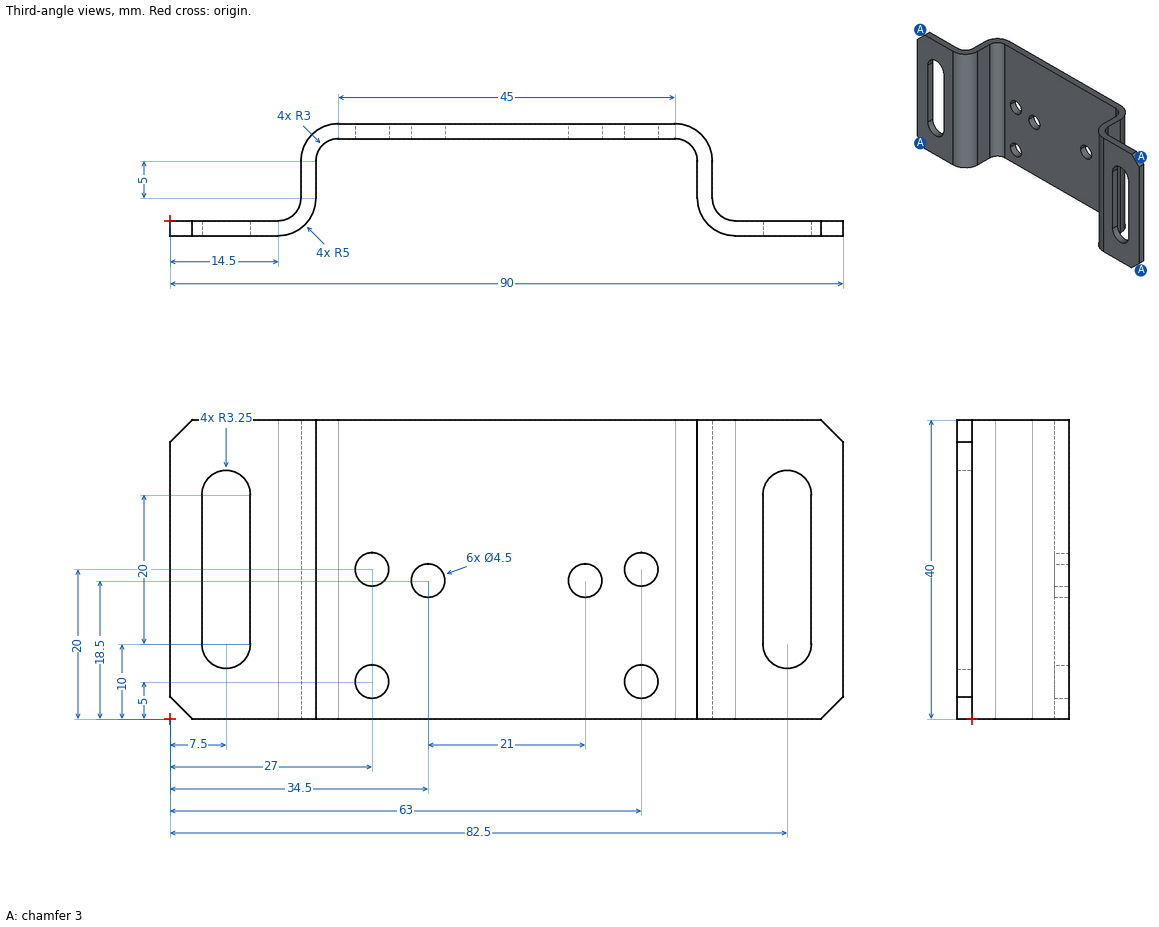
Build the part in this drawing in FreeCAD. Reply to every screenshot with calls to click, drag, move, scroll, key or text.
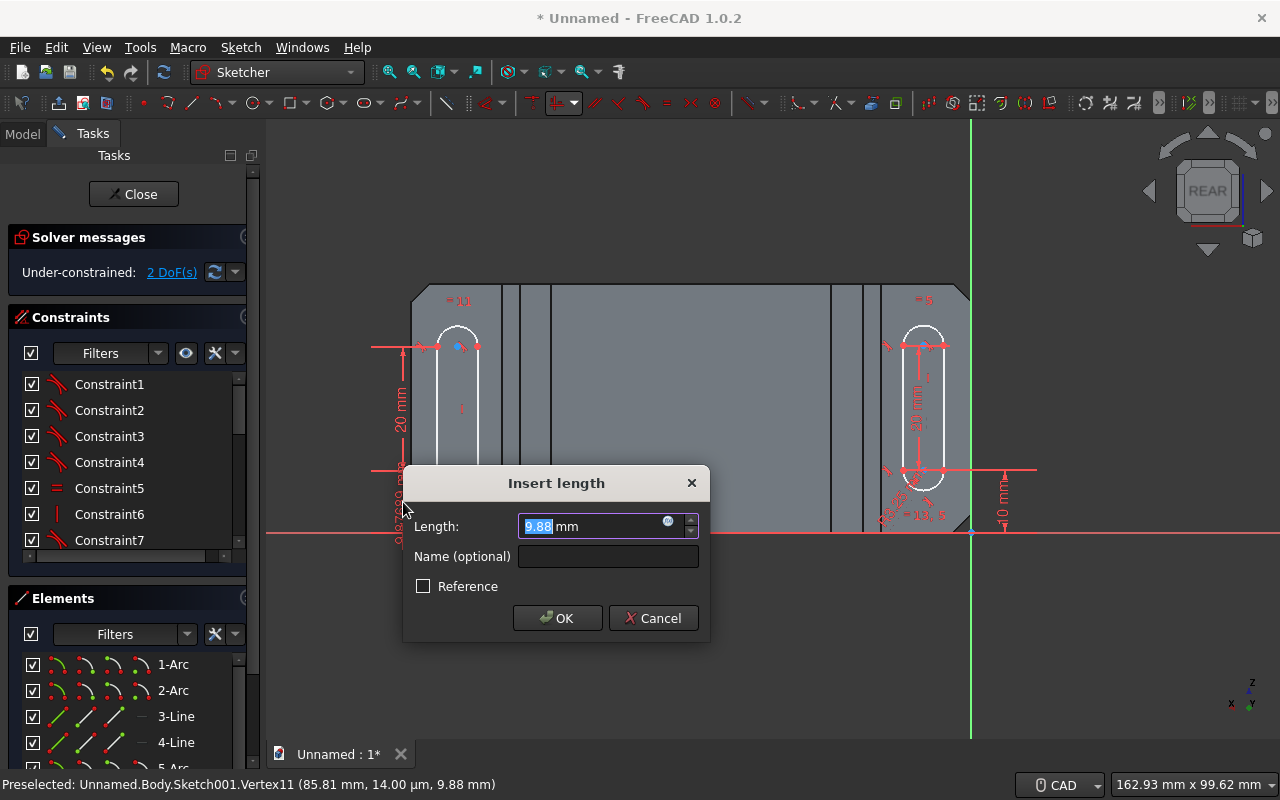
text(10)
key(Return)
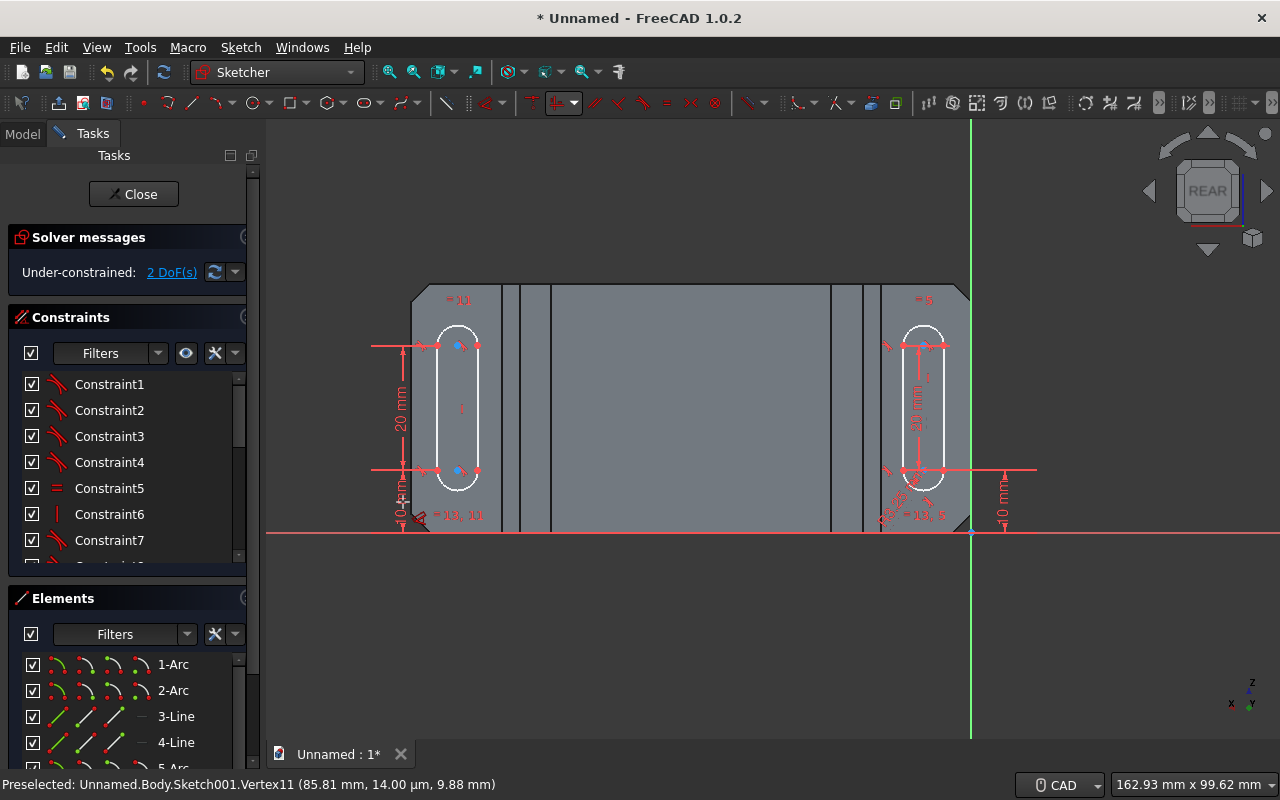
click(924, 470)
click(948, 567)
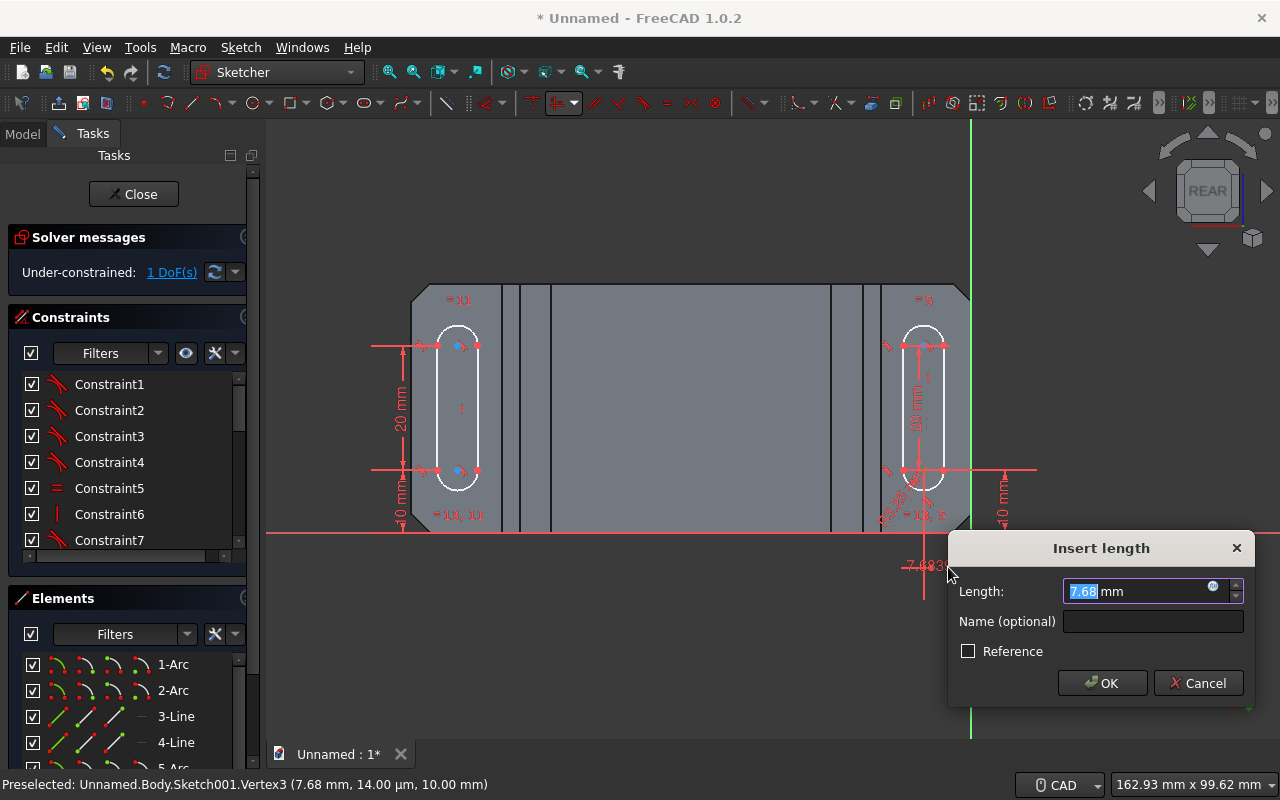
text(7.5)
key(Return)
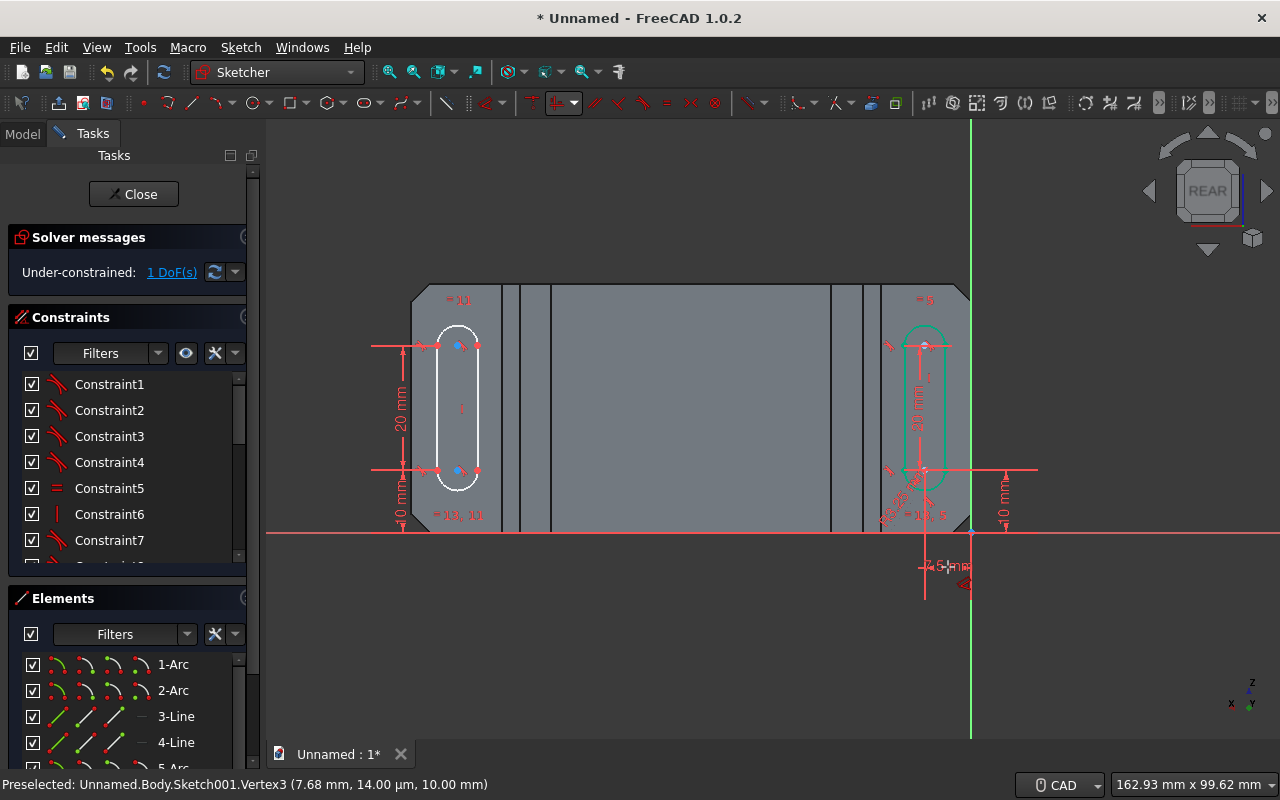
click(458, 470)
click(715, 567)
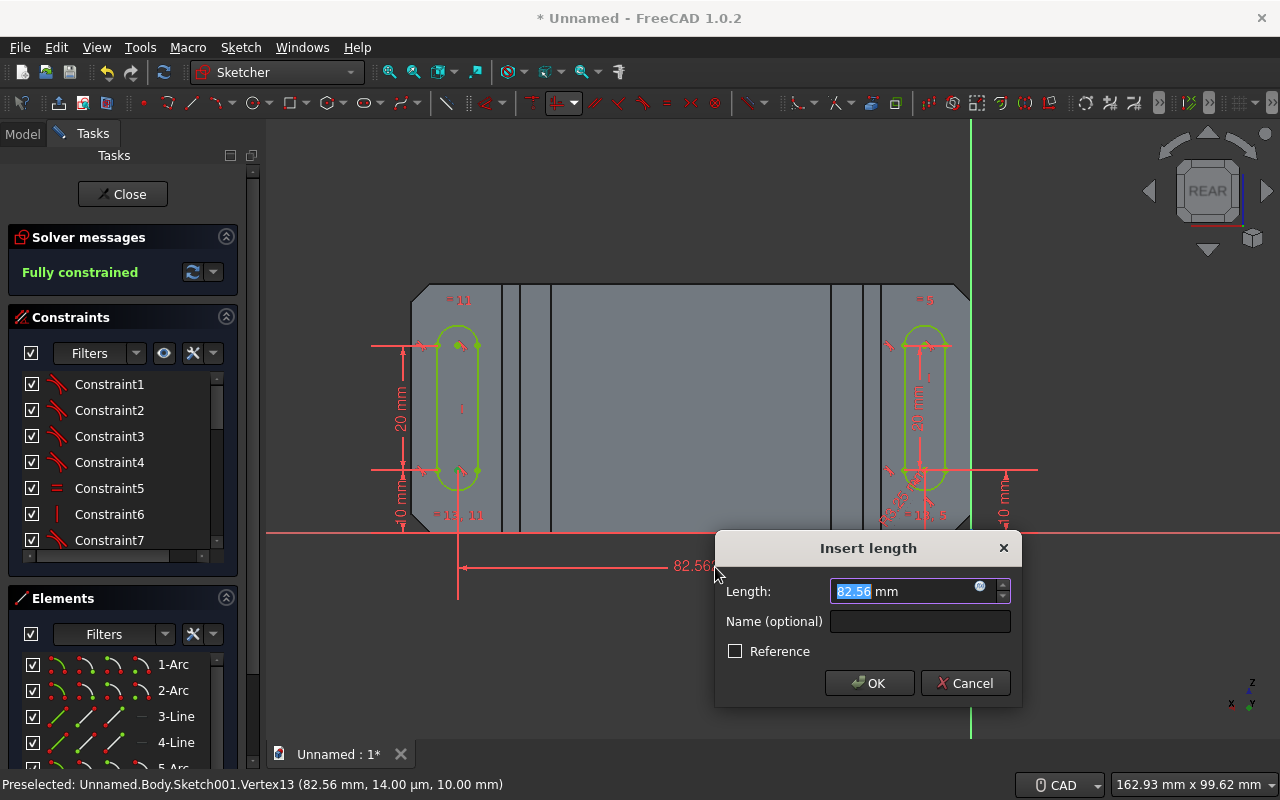
text(82.5)
key(Return)
key(Escape)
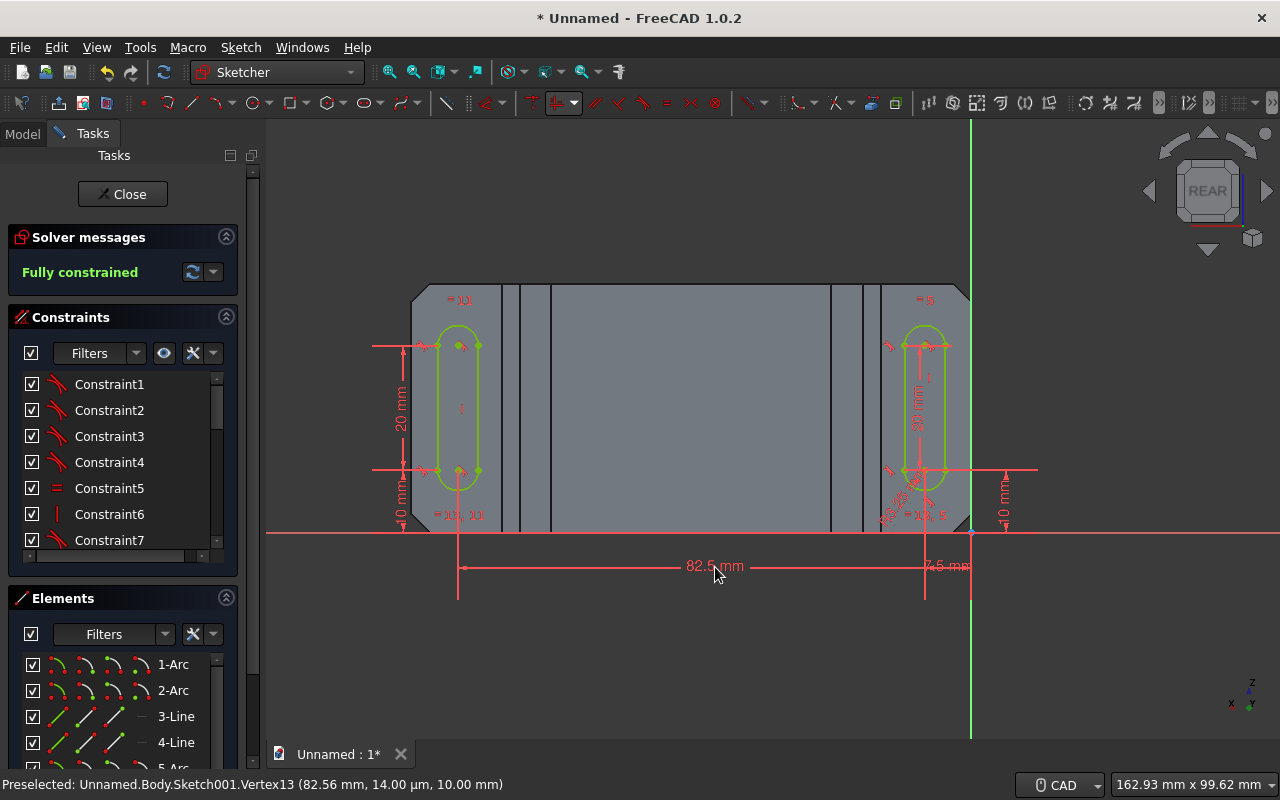
click(123, 194)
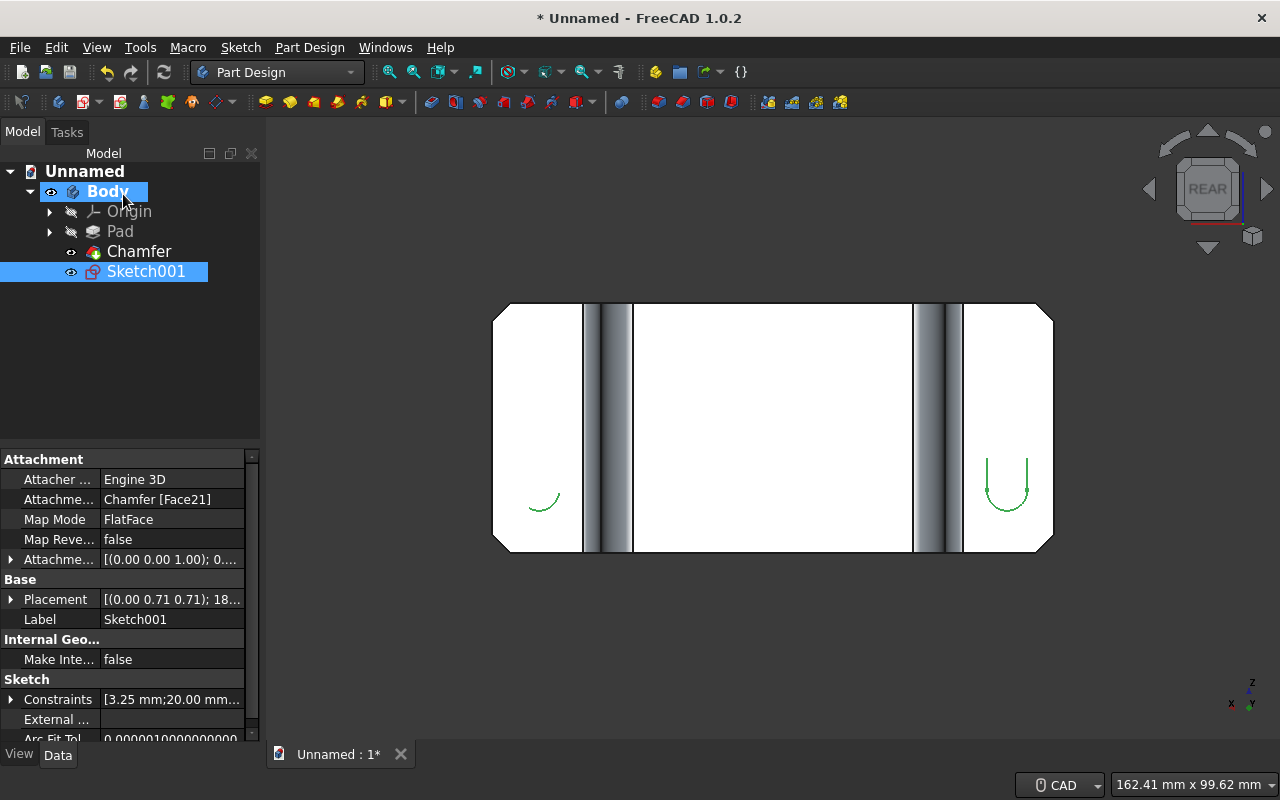
click(432, 102)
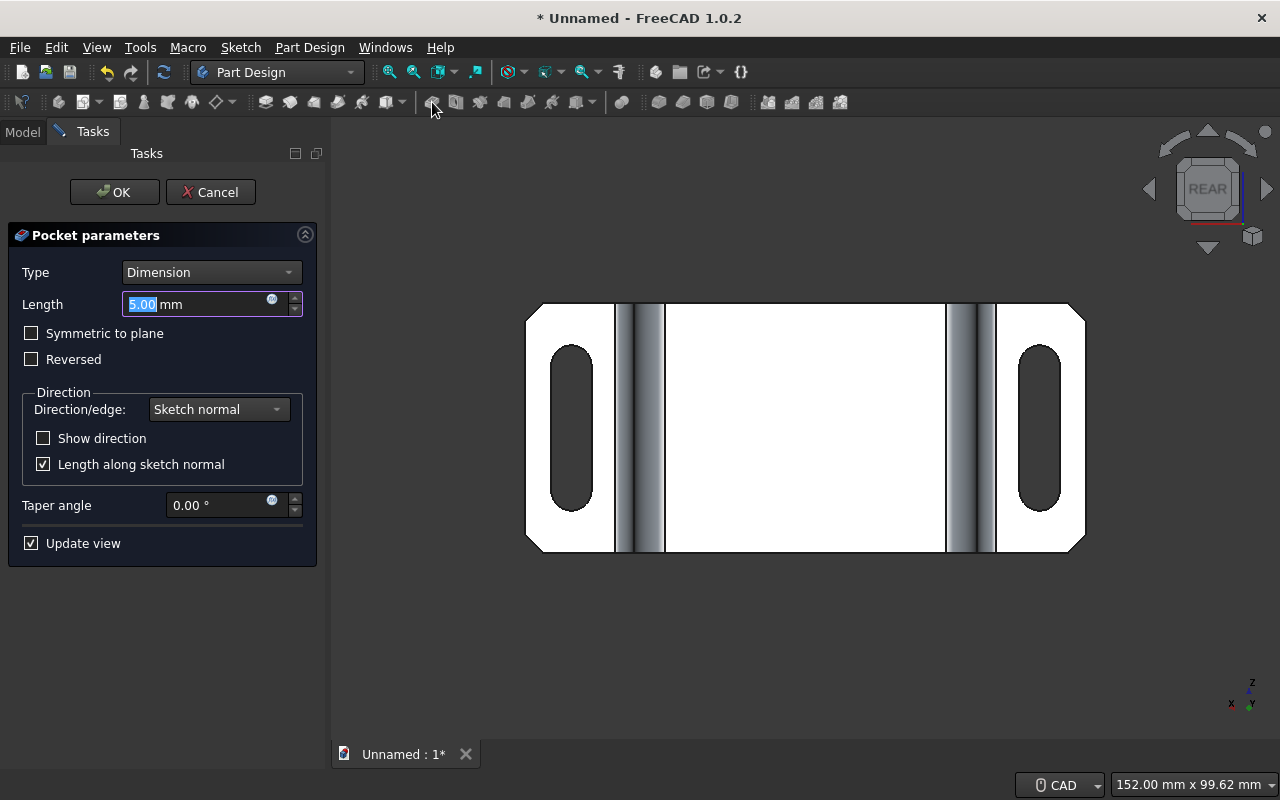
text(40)
key(Tab)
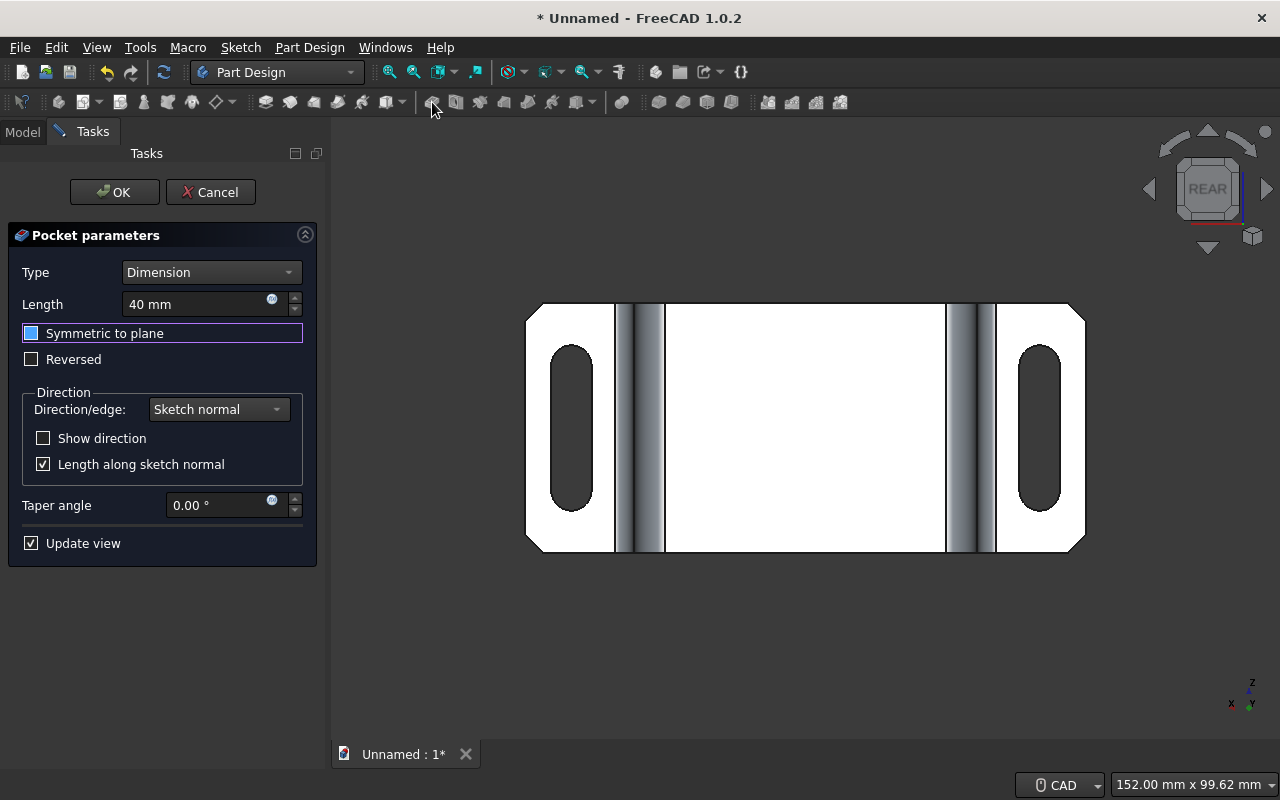
click(115, 192)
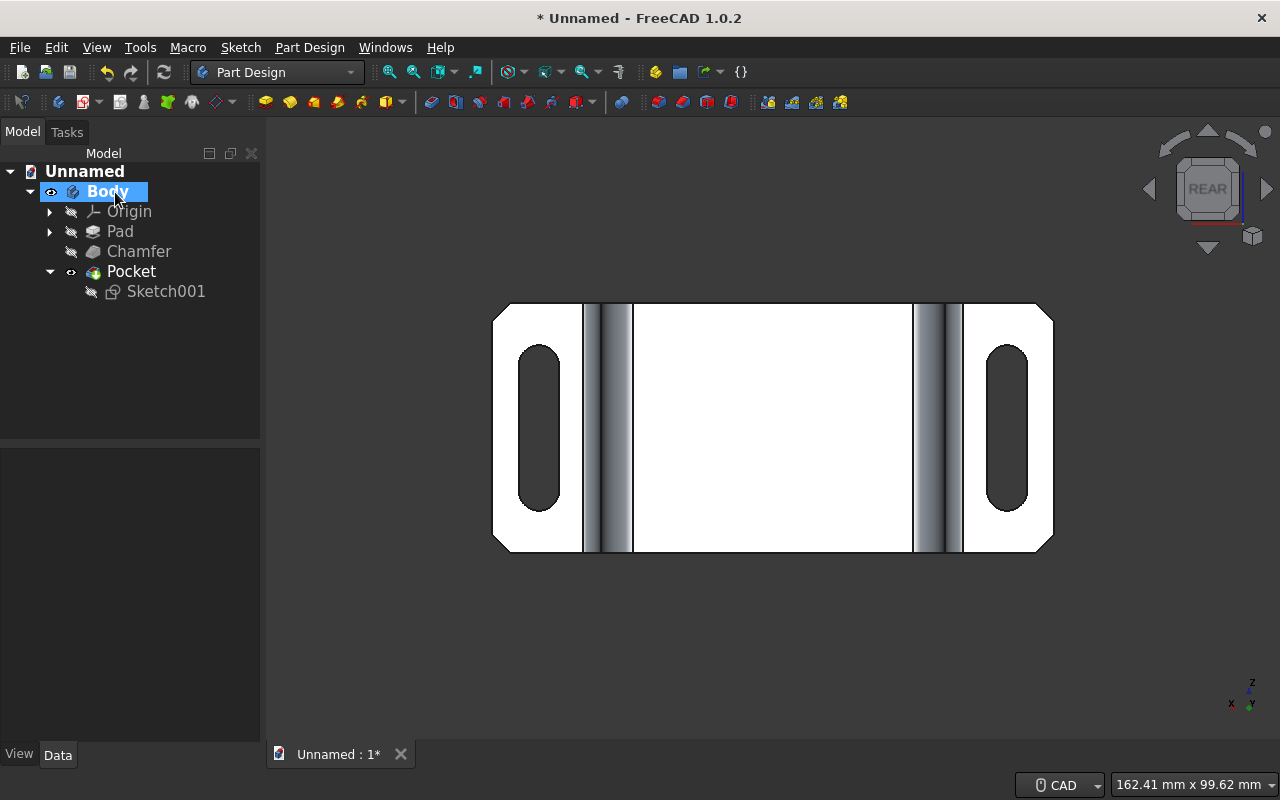
click(773, 427)